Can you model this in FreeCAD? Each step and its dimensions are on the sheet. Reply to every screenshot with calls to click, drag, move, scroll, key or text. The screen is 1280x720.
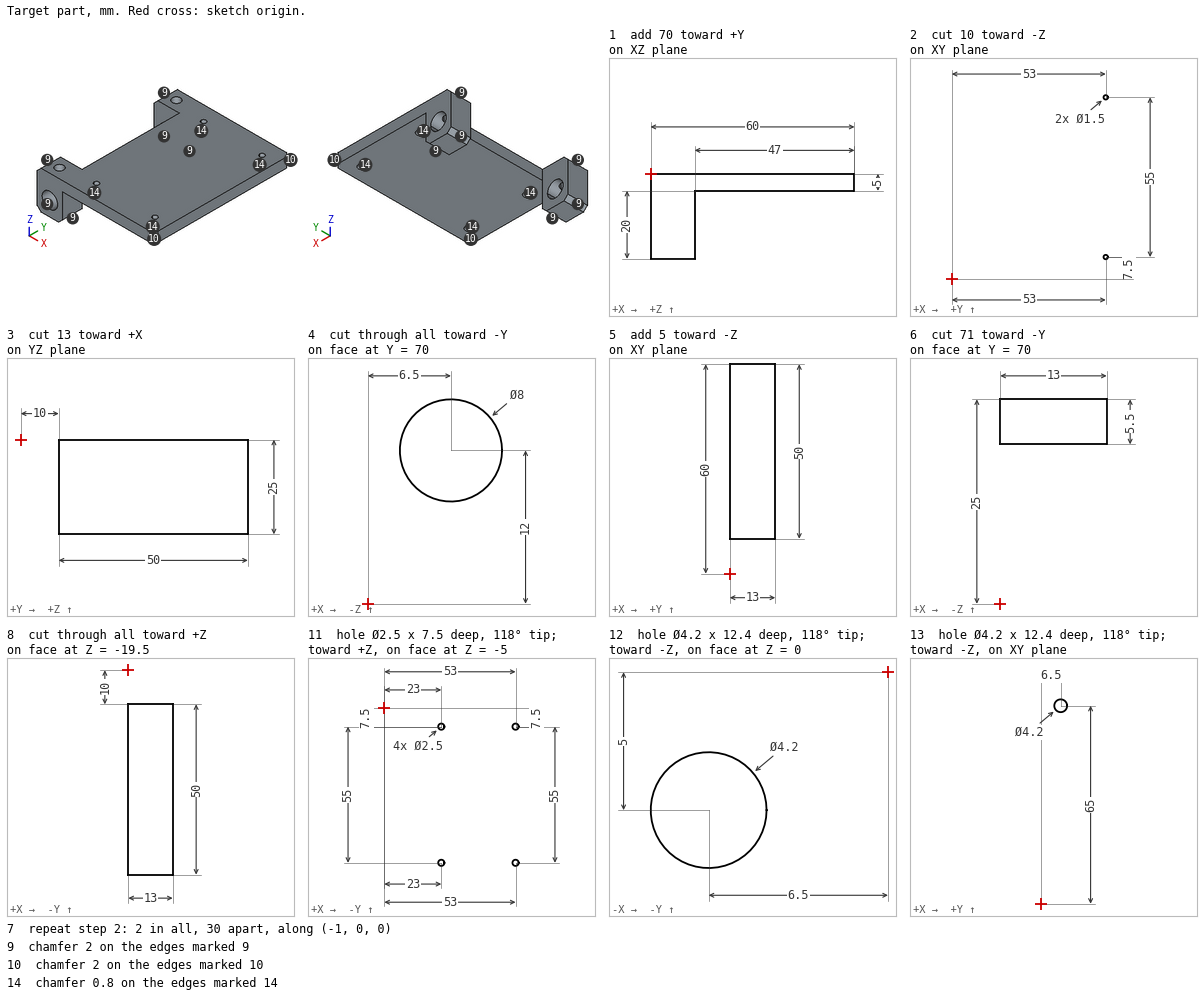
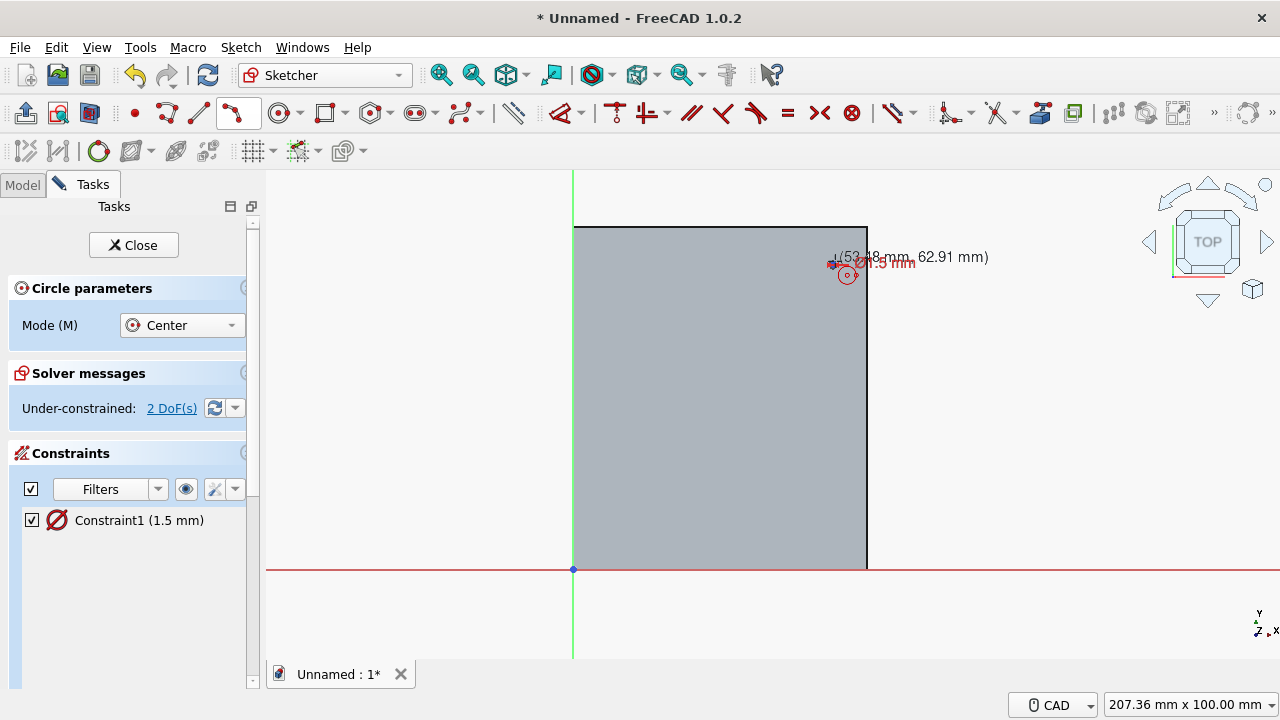
scroll(833, 533, up, 10)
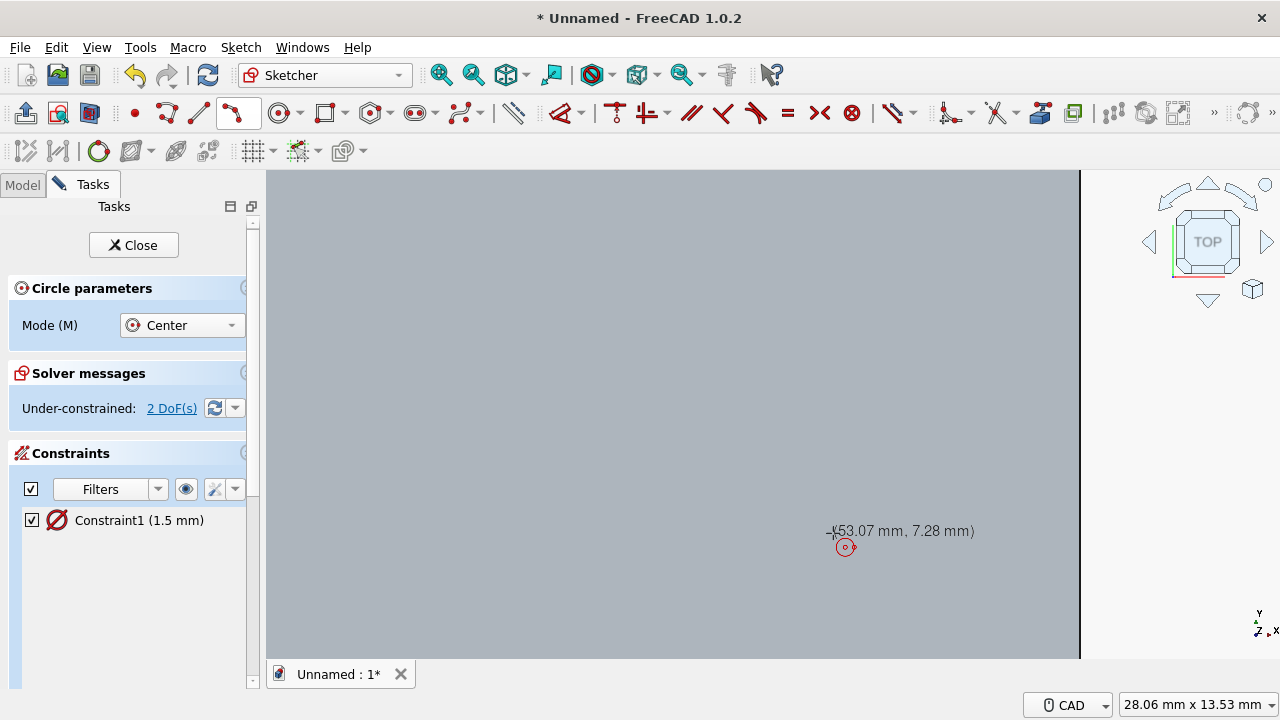
scroll(833, 533, down, 10)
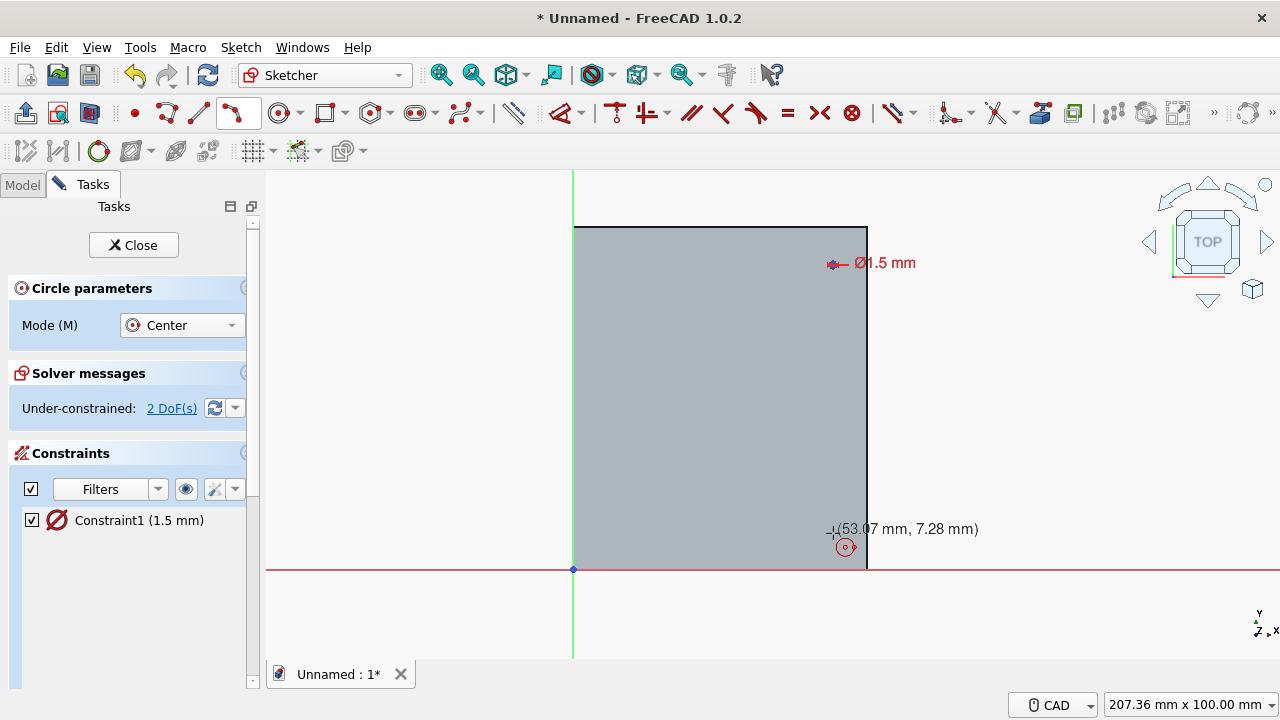
click(833, 533)
move(835, 530)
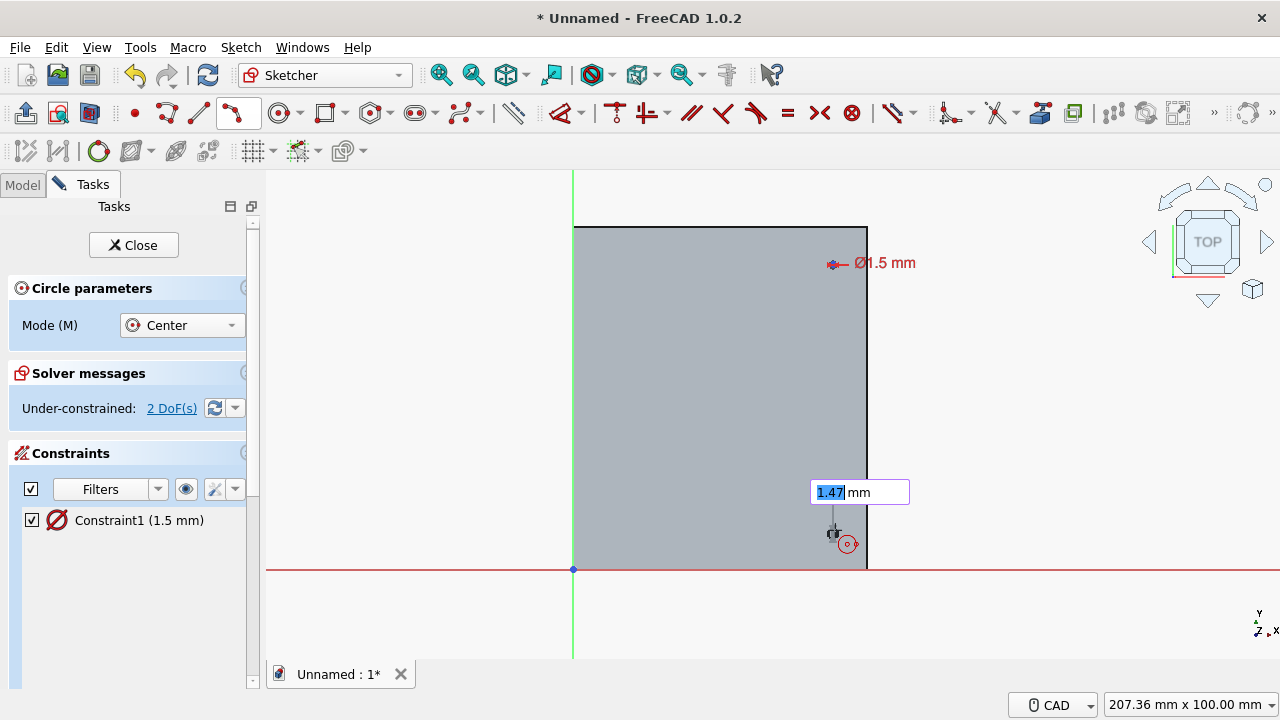
text(1.5)
key(Return)
key(Escape)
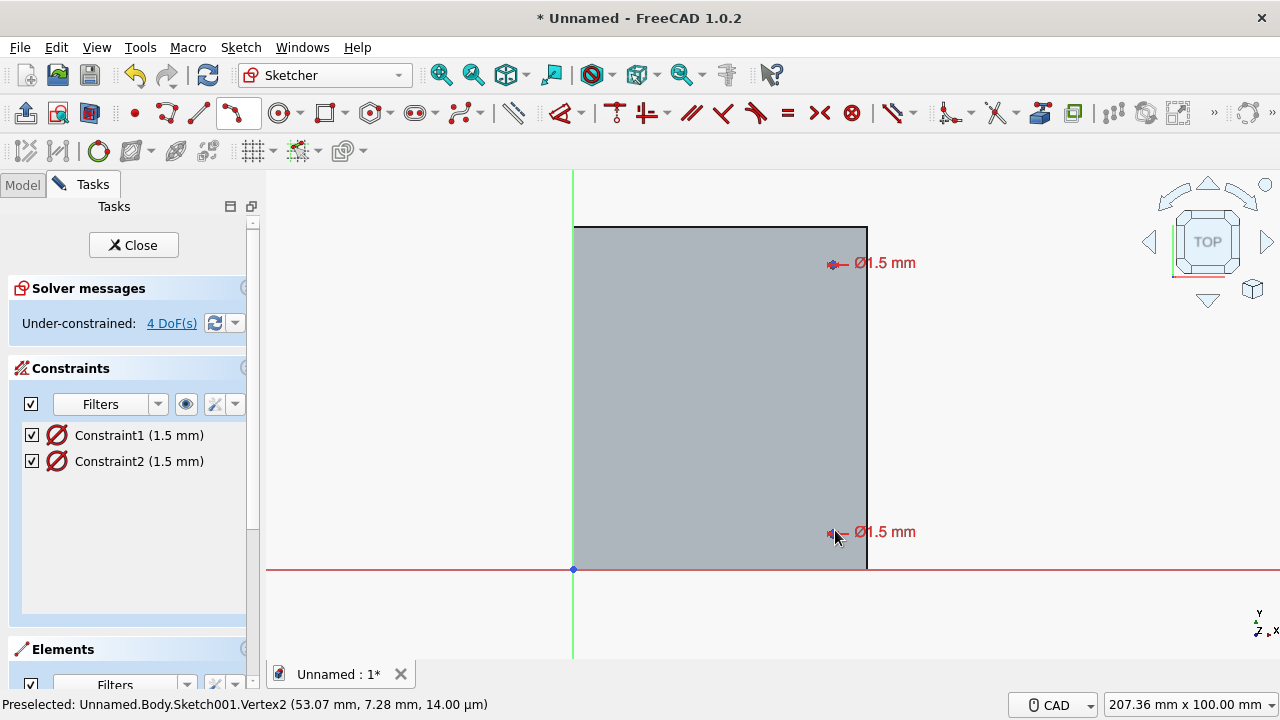
key(d)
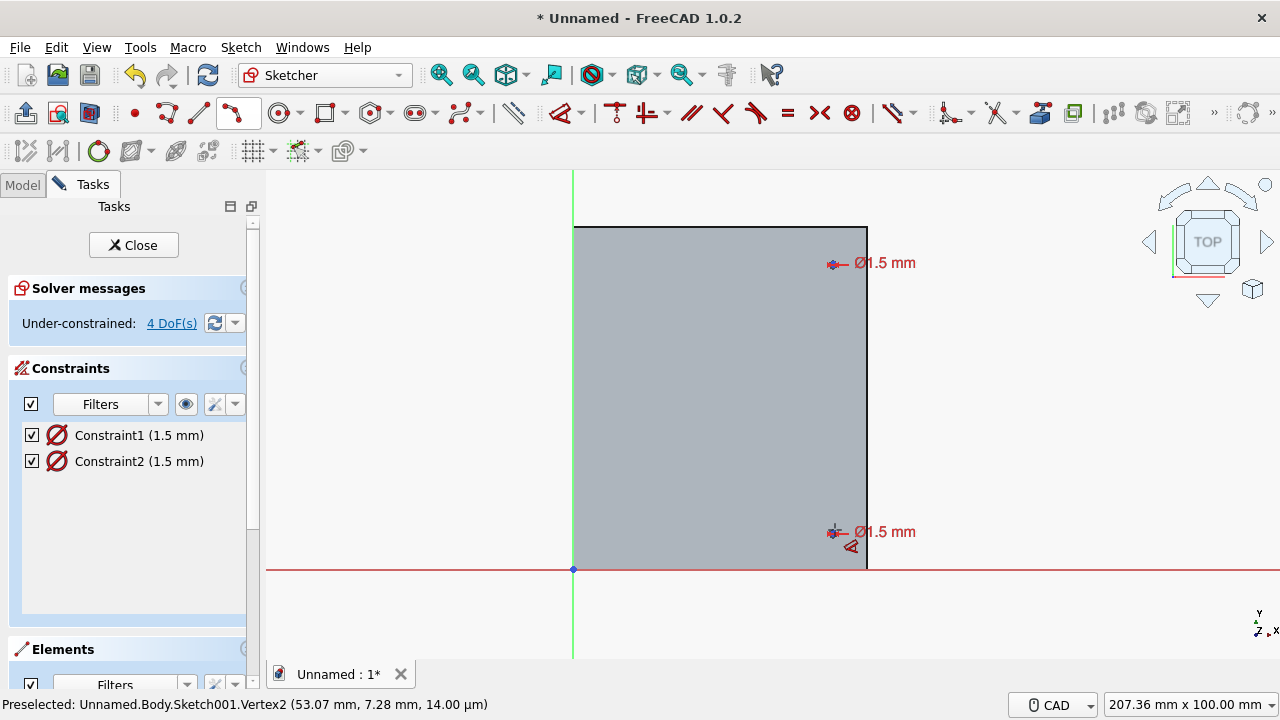
click(833, 265)
click(703, 604)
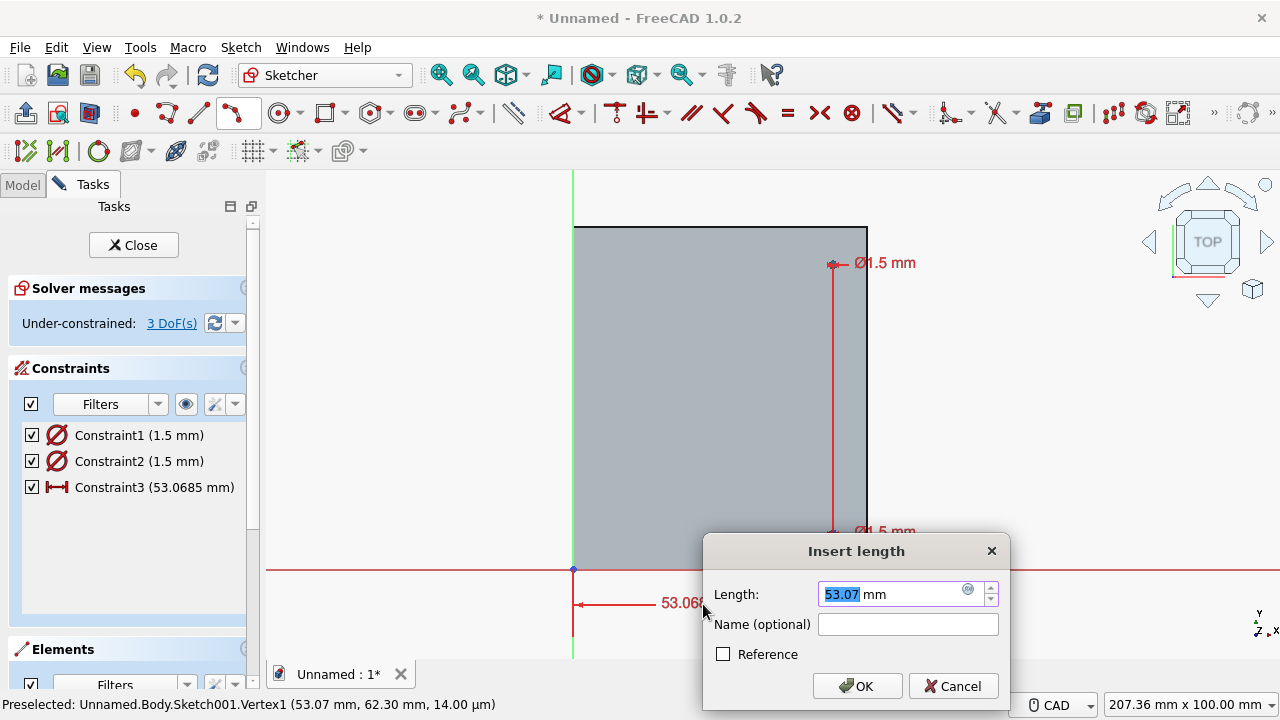
text(53)
key(Return)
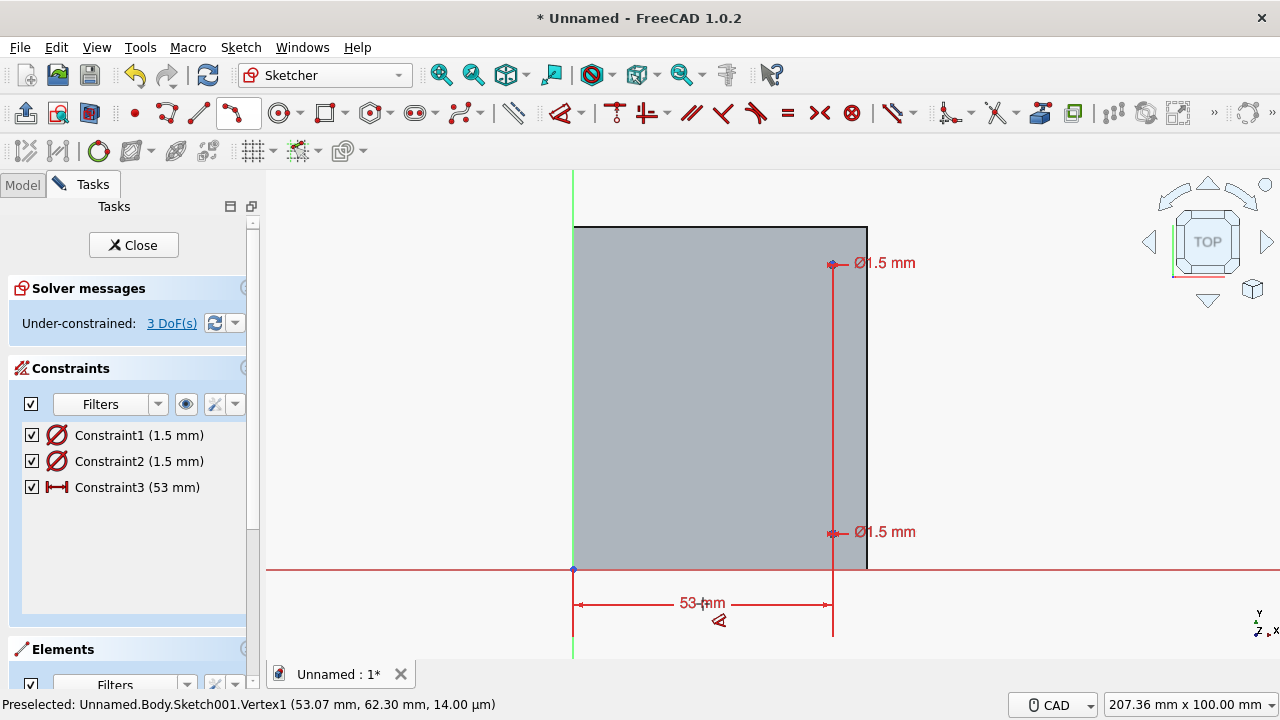
click(833, 534)
click(612, 604)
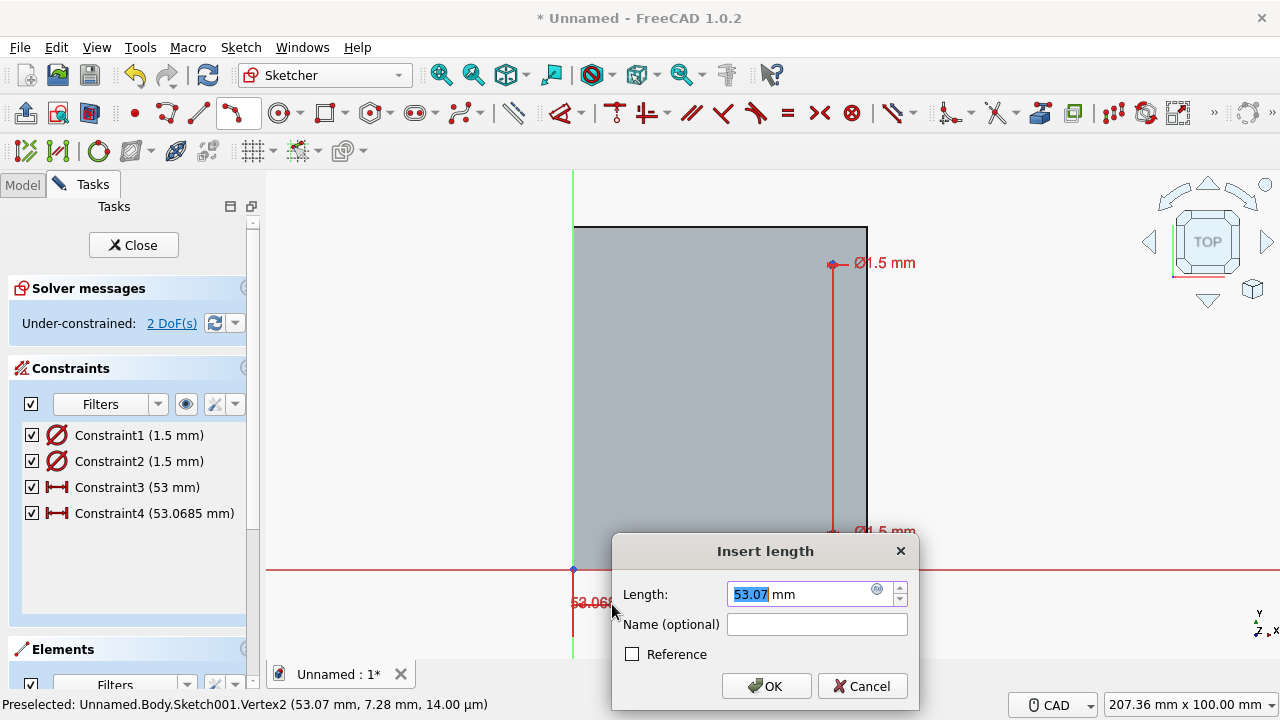
text(53)
key(Return)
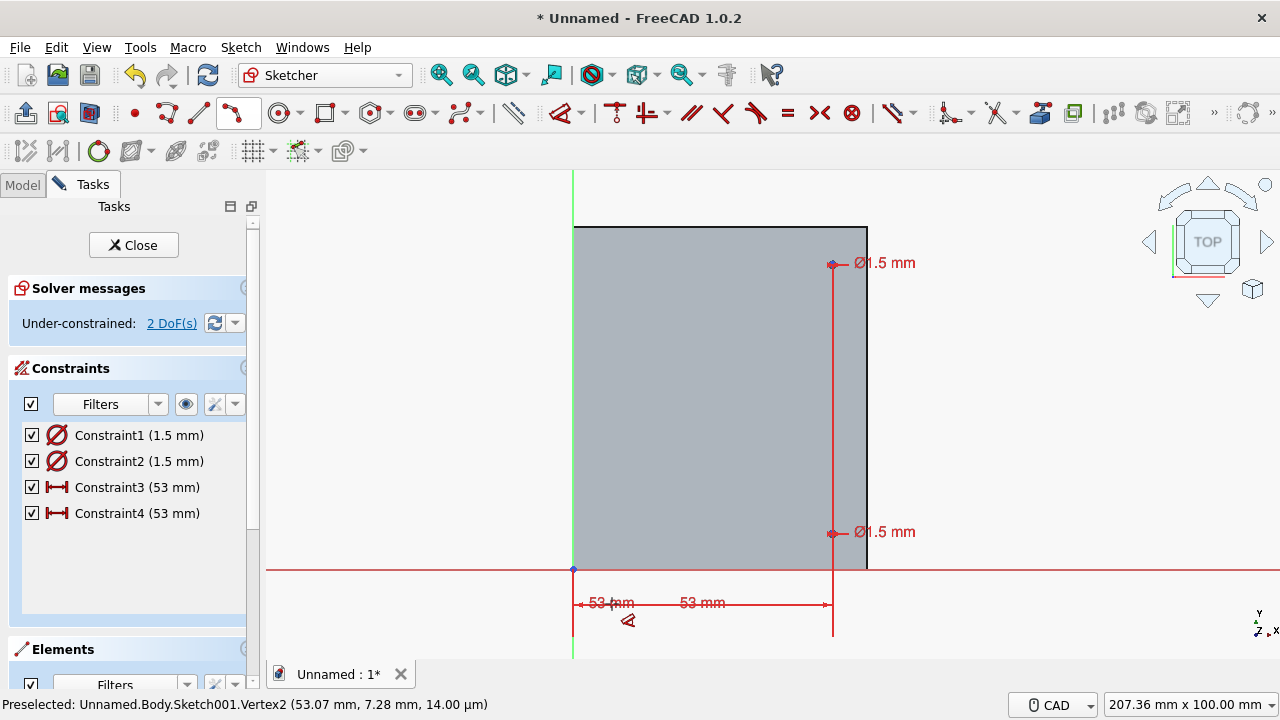
click(833, 534)
click(539, 552)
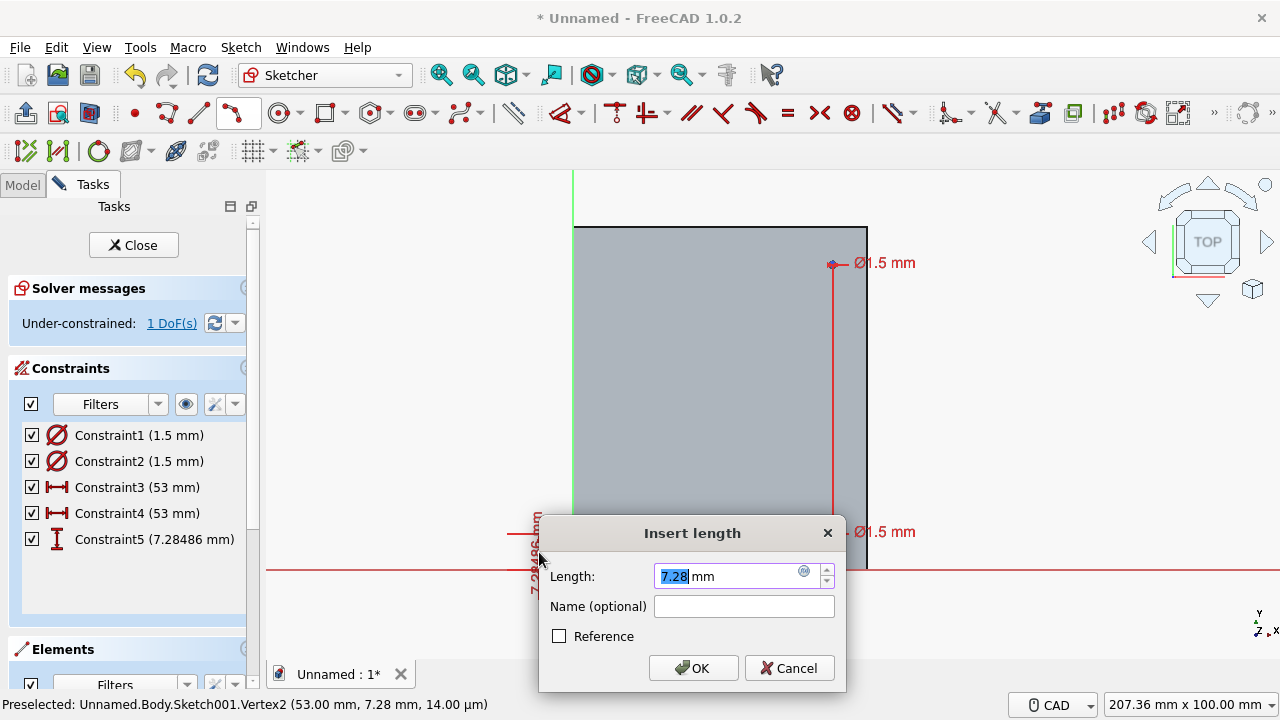
text(7.5)
key(Return)